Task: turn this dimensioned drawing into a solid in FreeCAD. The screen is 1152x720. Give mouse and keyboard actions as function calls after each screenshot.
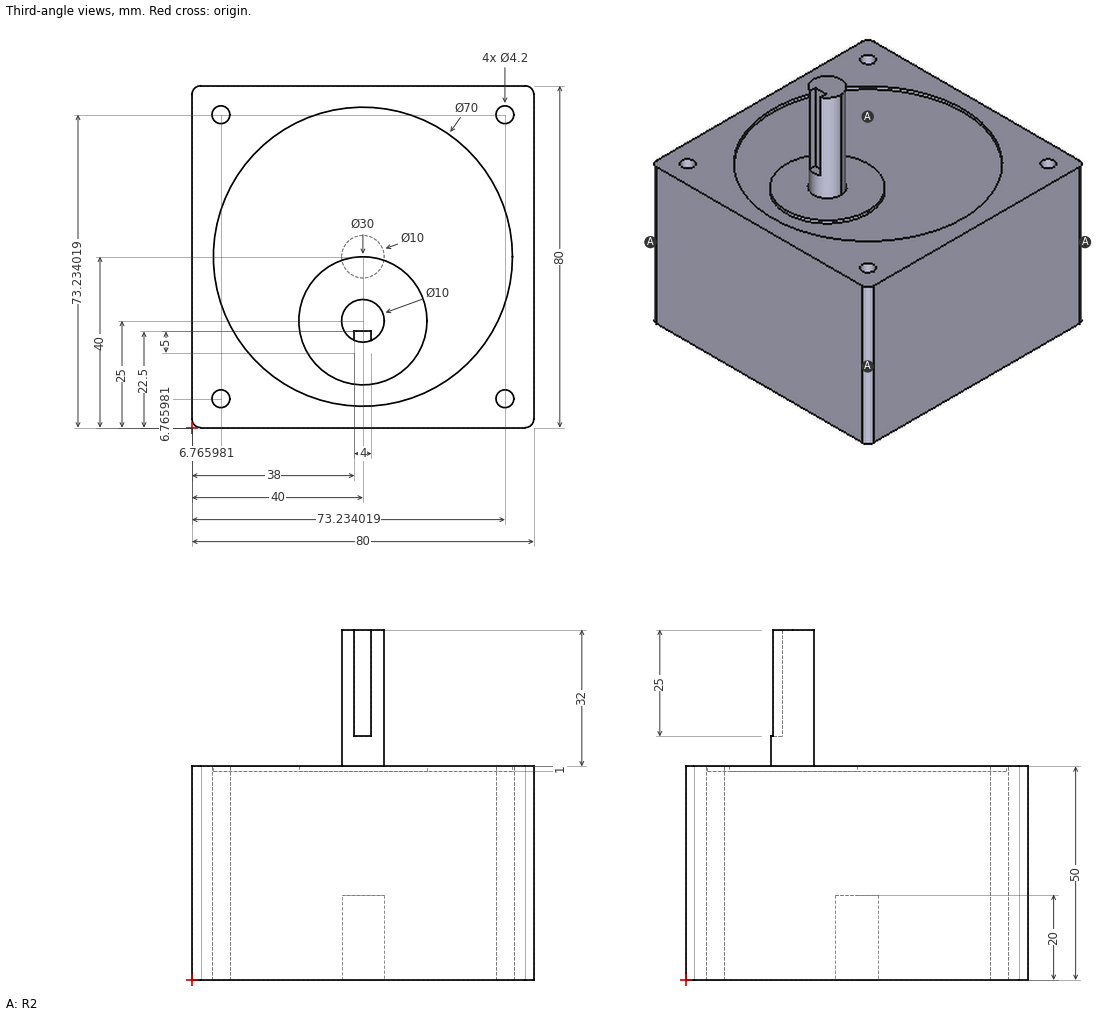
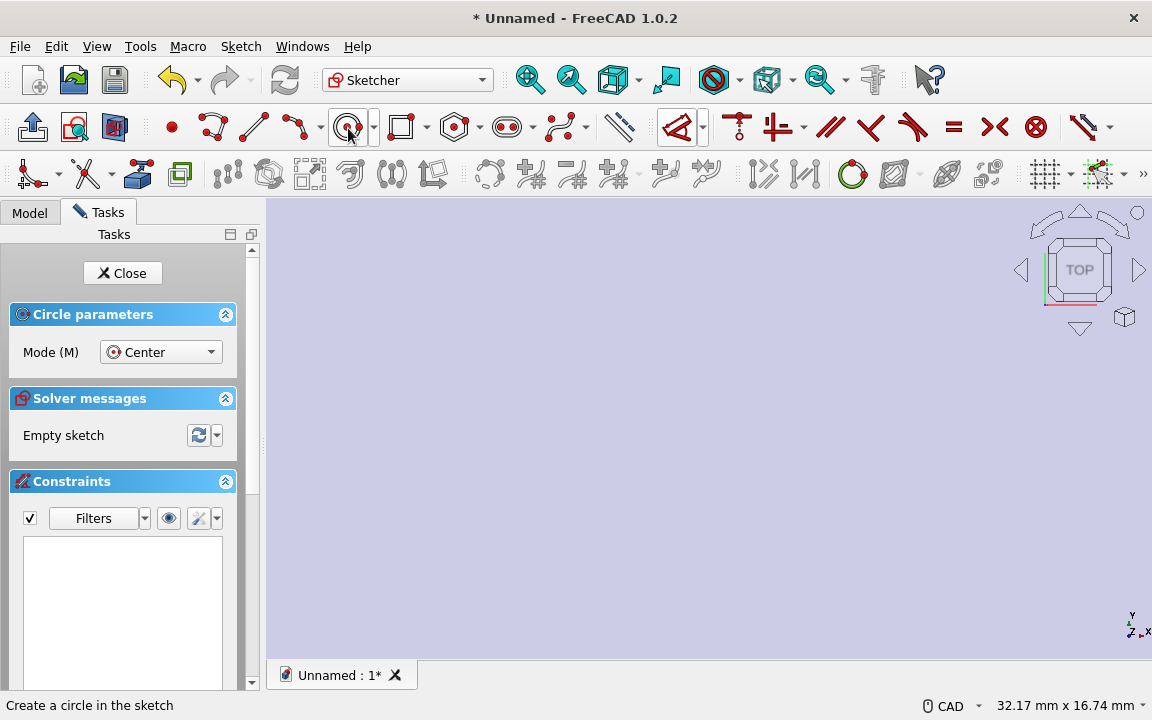
click(635, 428)
click(733, 331)
key(Escape)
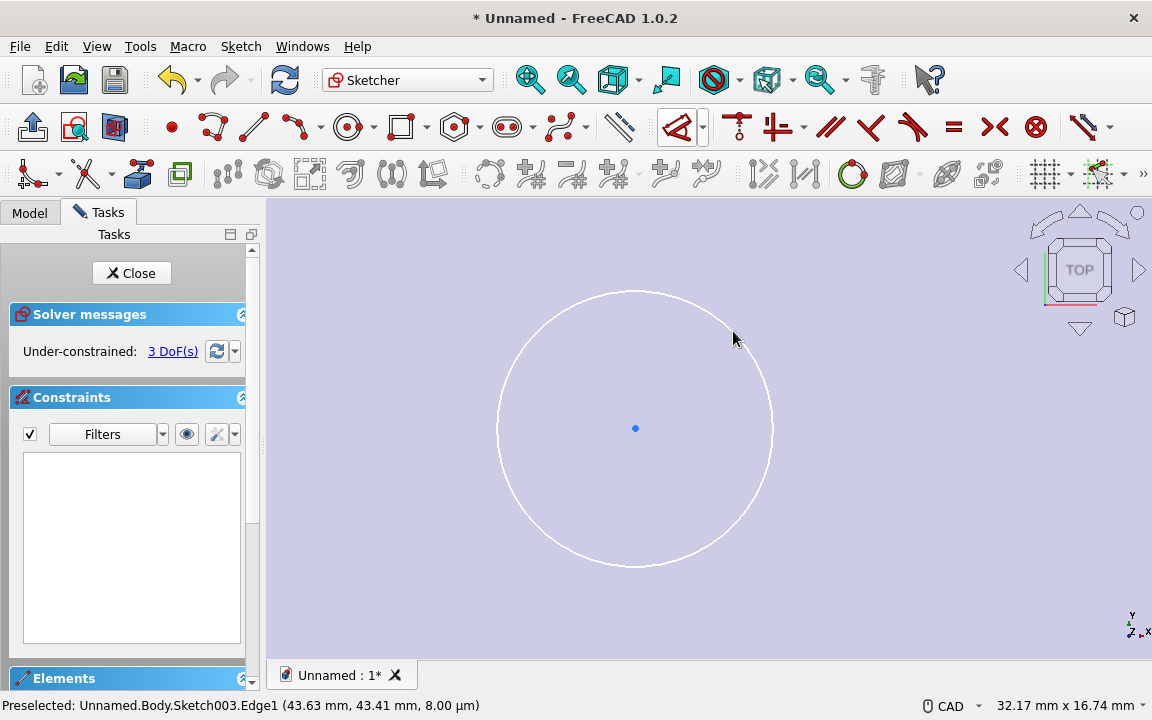
click(732, 331)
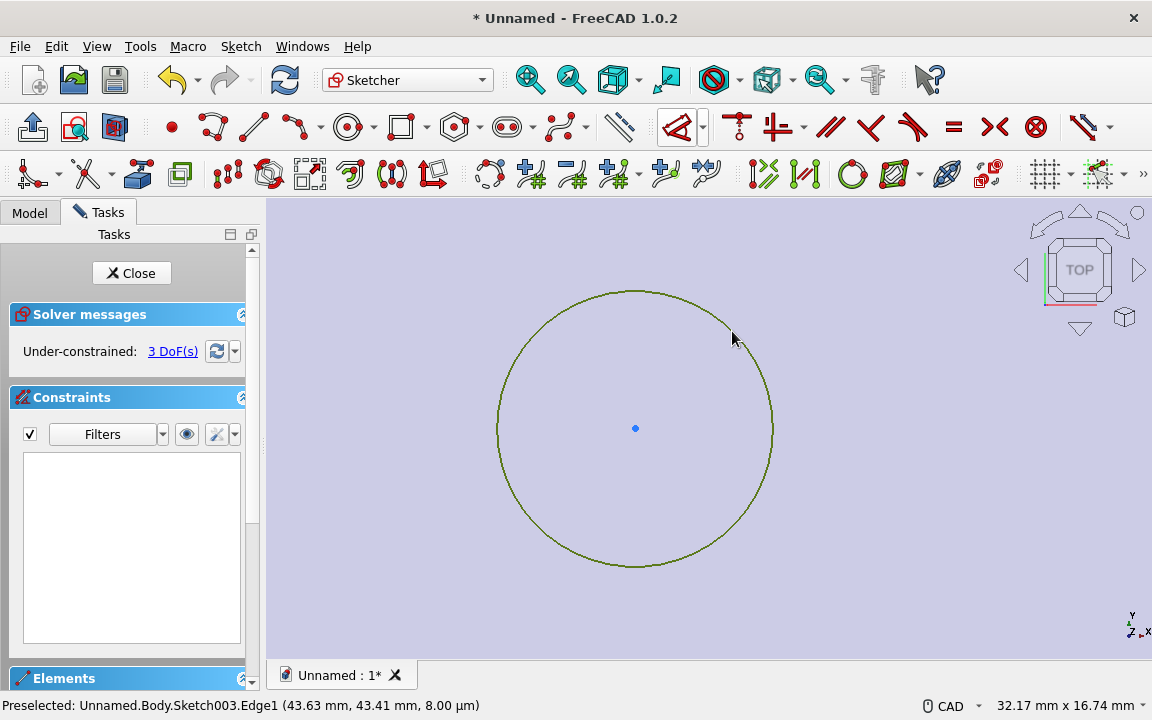
click(702, 128)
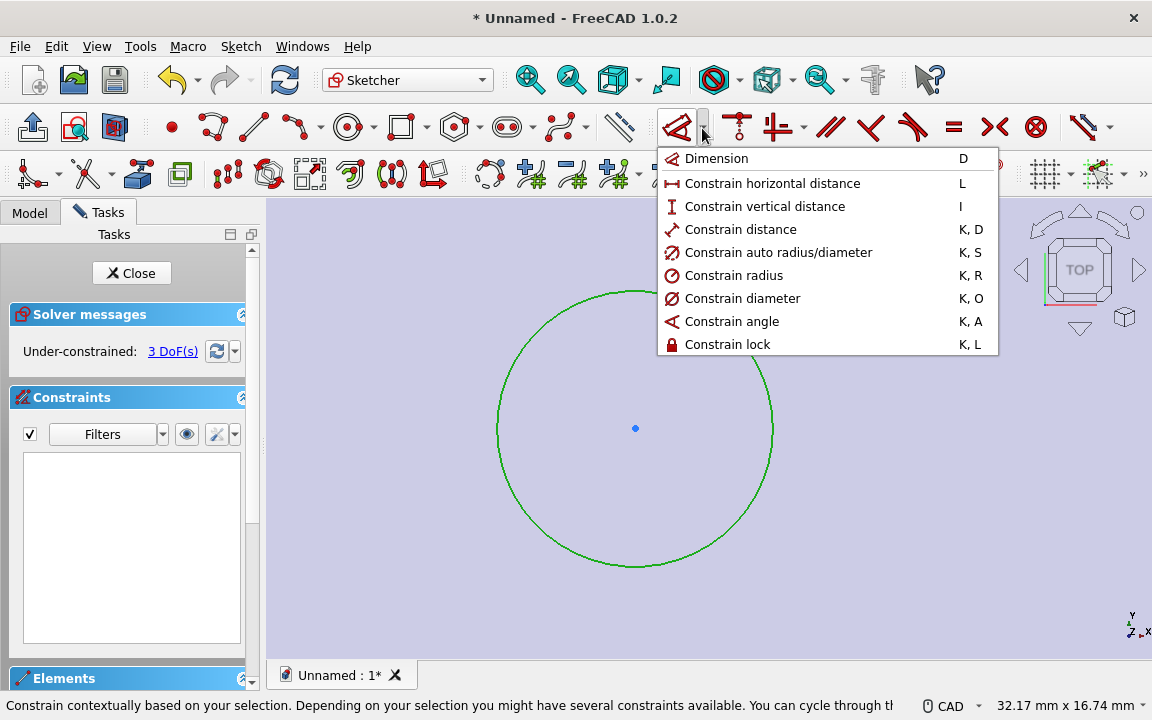
click(828, 298)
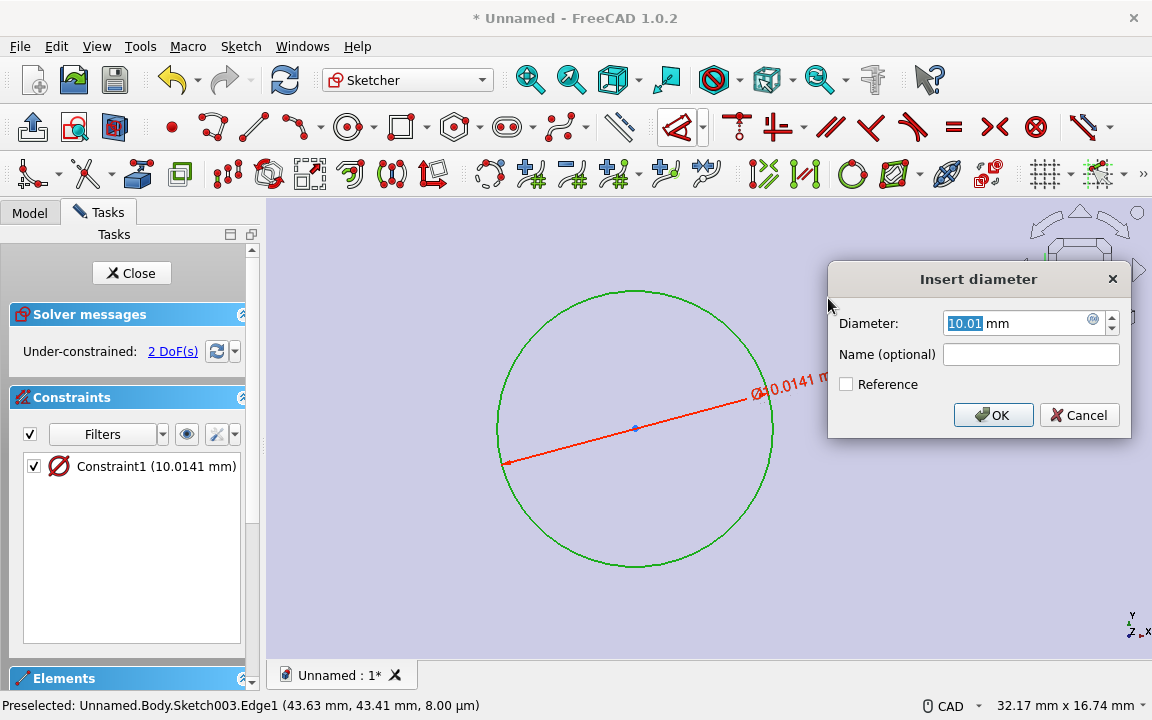
text(10)
key(Return)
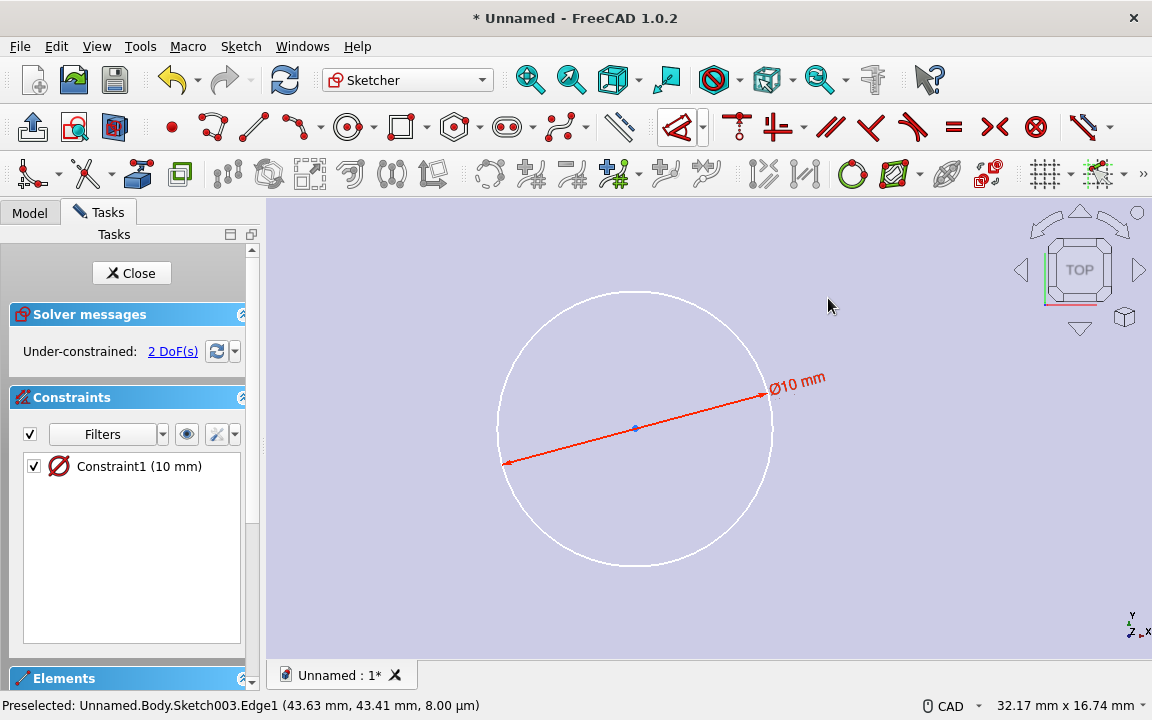
click(635, 429)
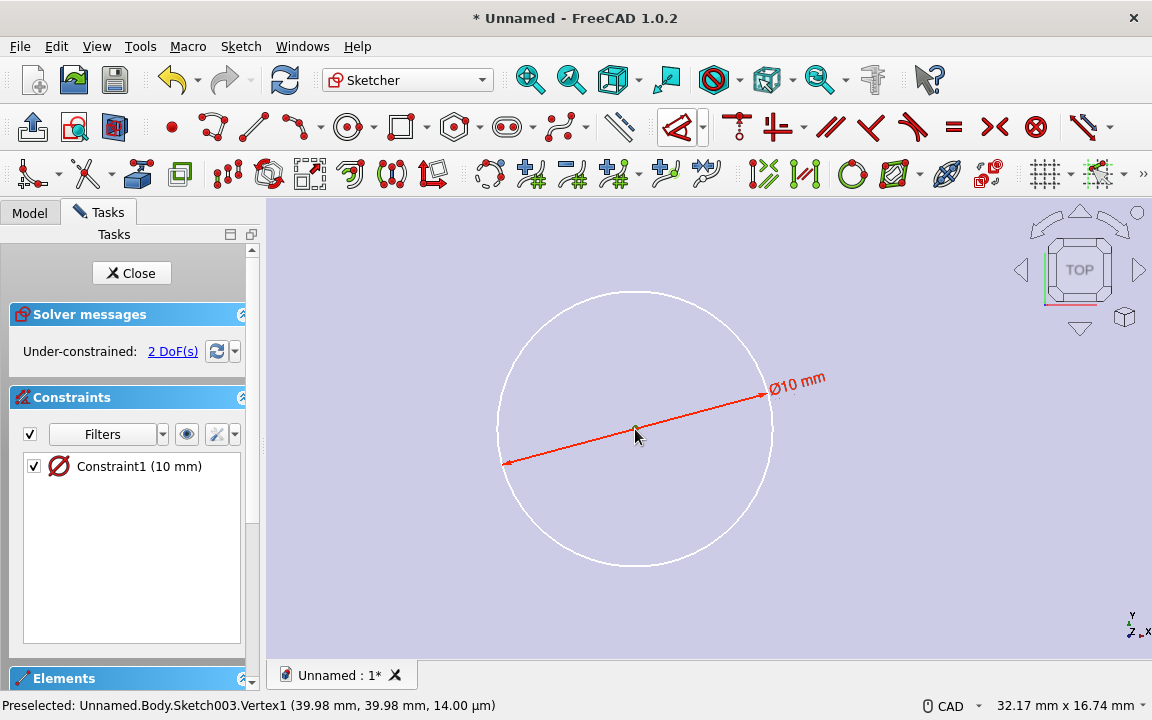
click(702, 128)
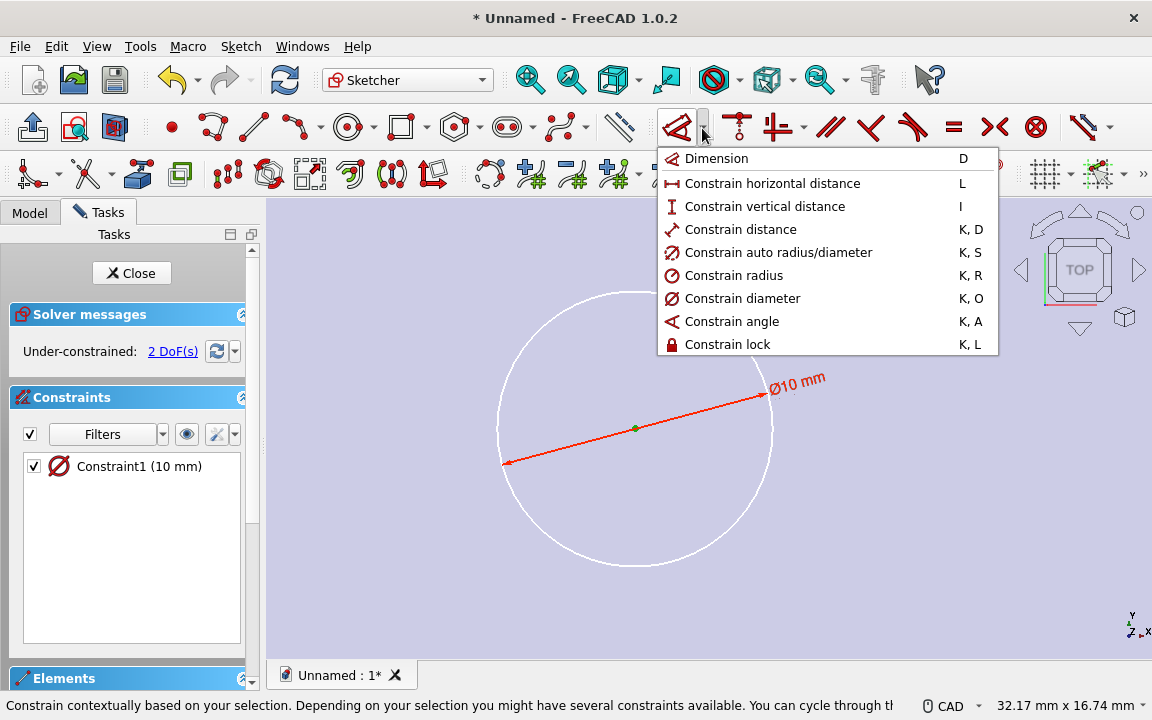
click(828, 184)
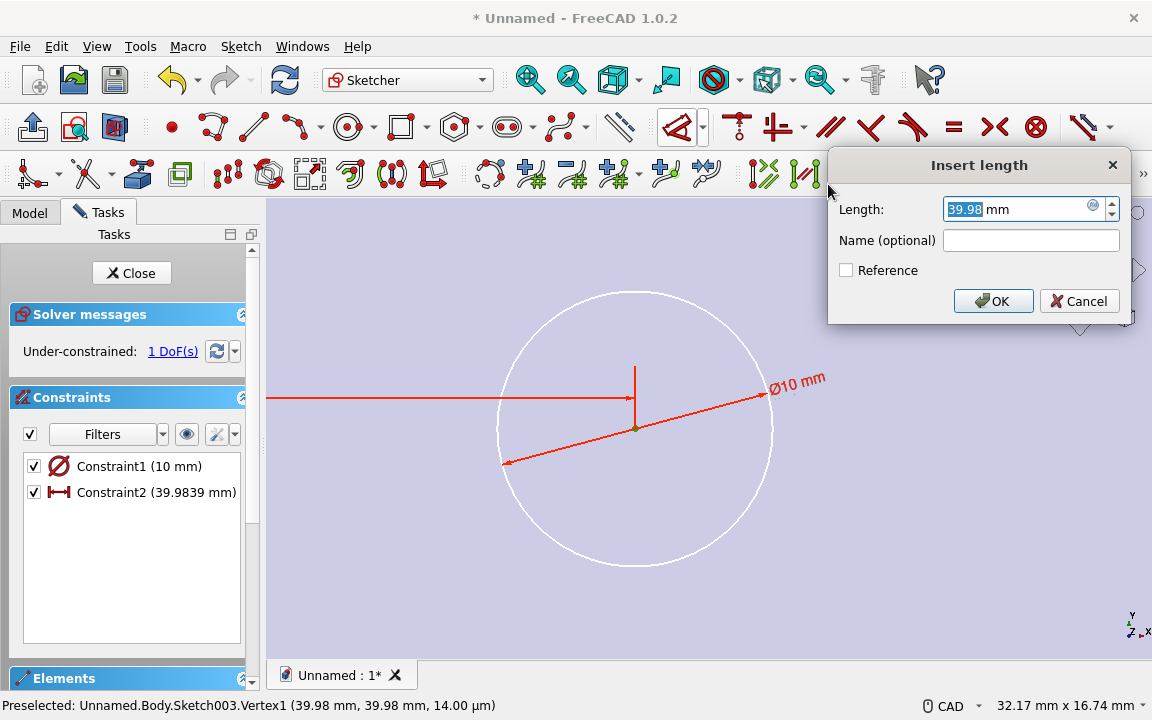
text(40)
key(Return)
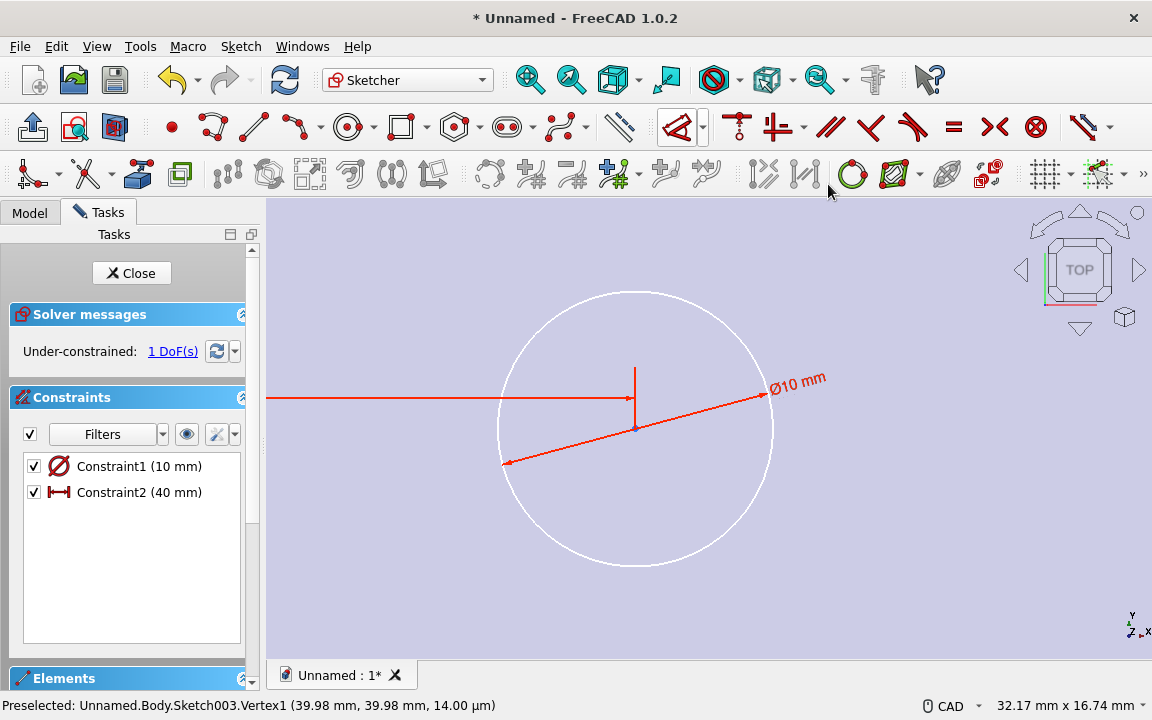
click(635, 429)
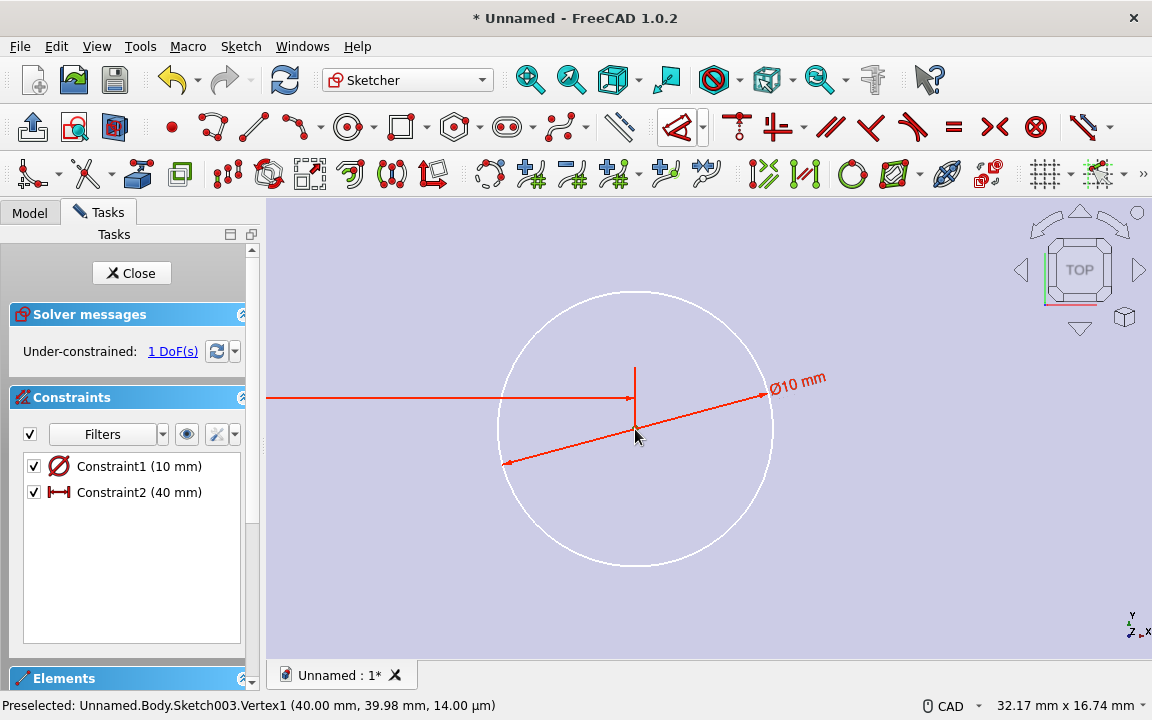
key(i)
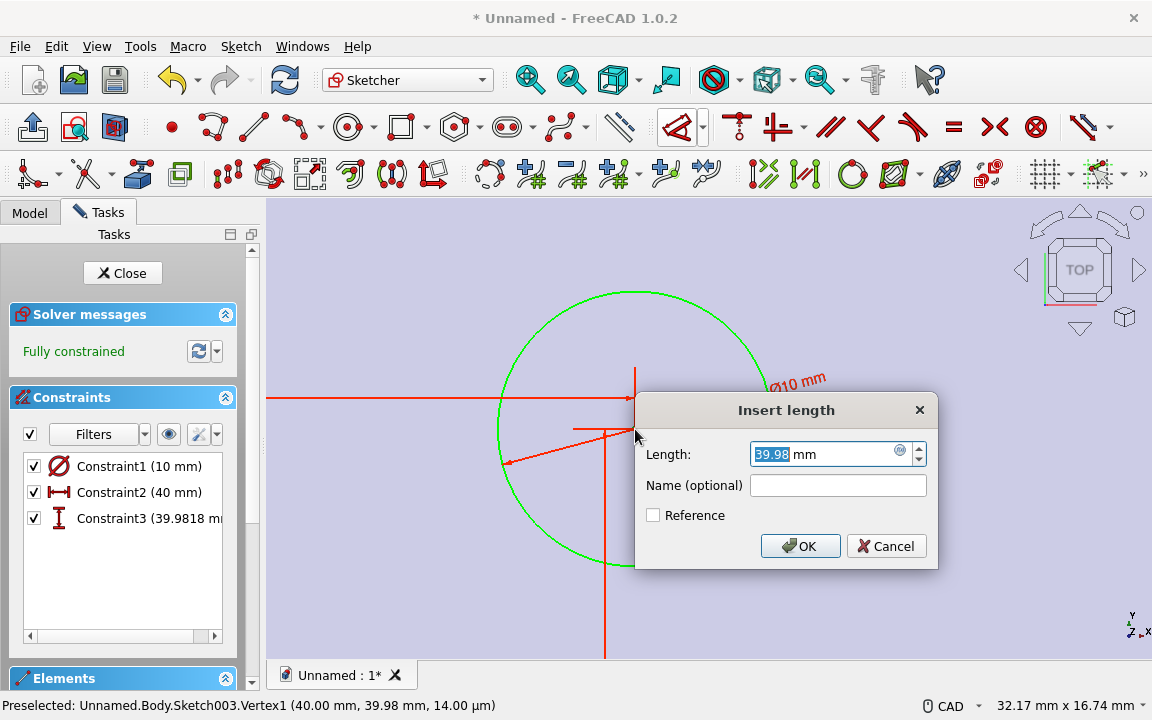
text(40)
key(Return)